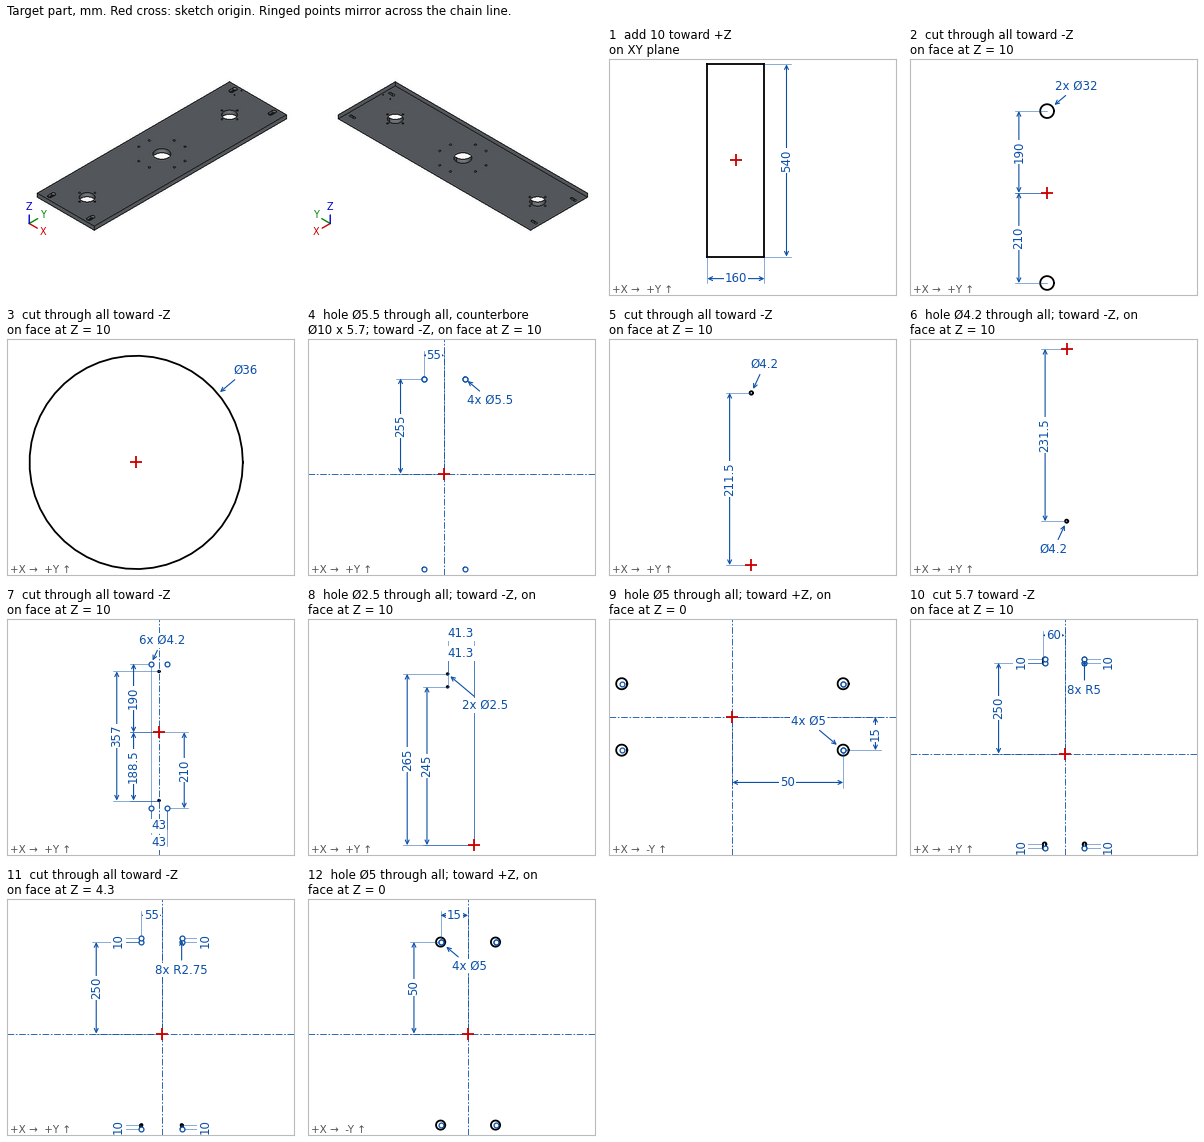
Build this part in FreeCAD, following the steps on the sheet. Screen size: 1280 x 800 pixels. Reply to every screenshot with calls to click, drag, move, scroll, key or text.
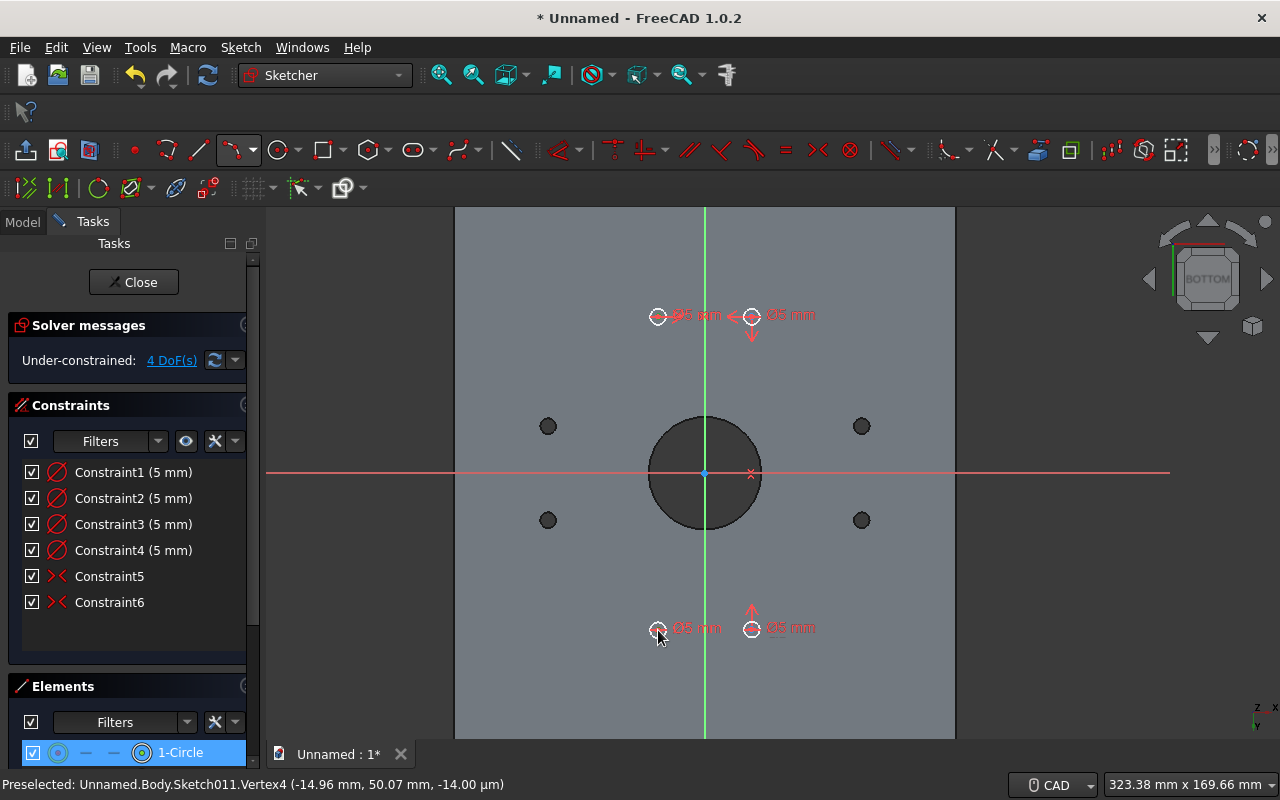
click(353, 473)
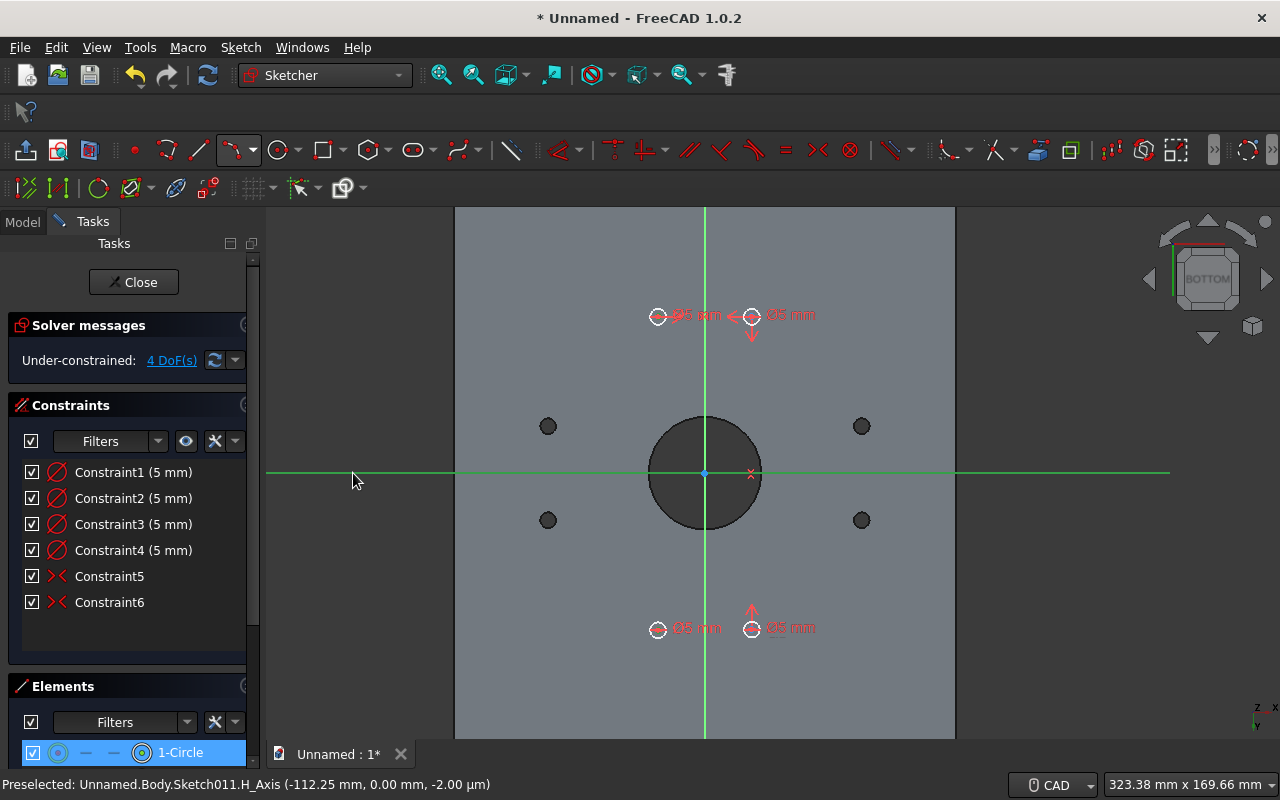
key(s)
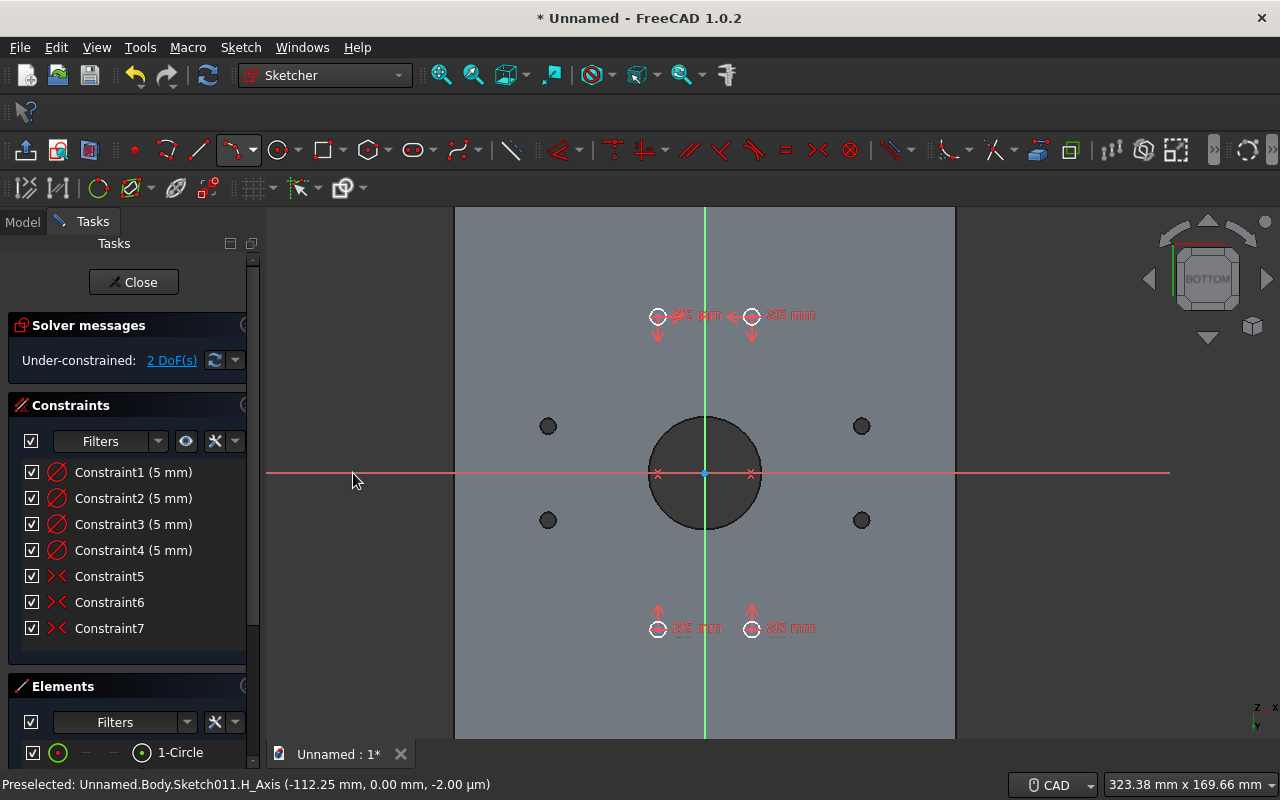
click(558, 150)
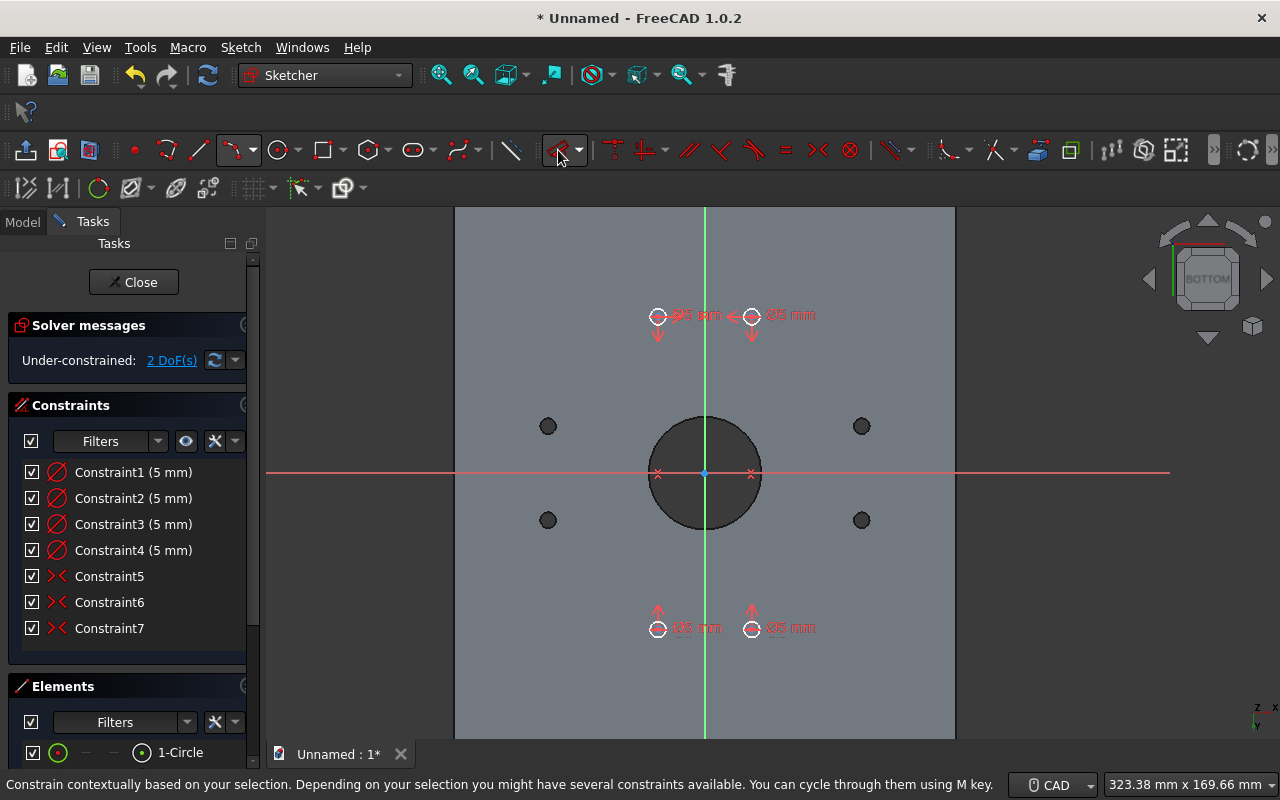
click(658, 317)
click(682, 283)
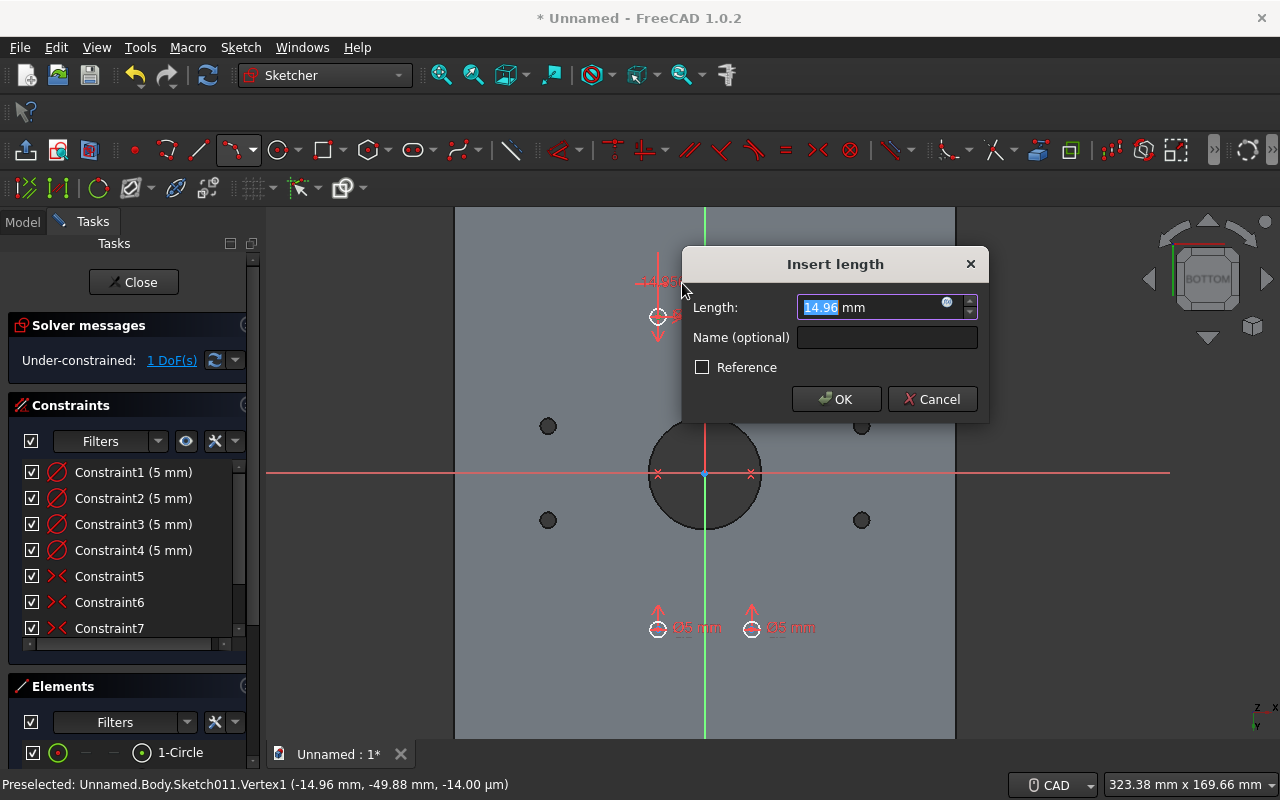
text(15)
key(Return)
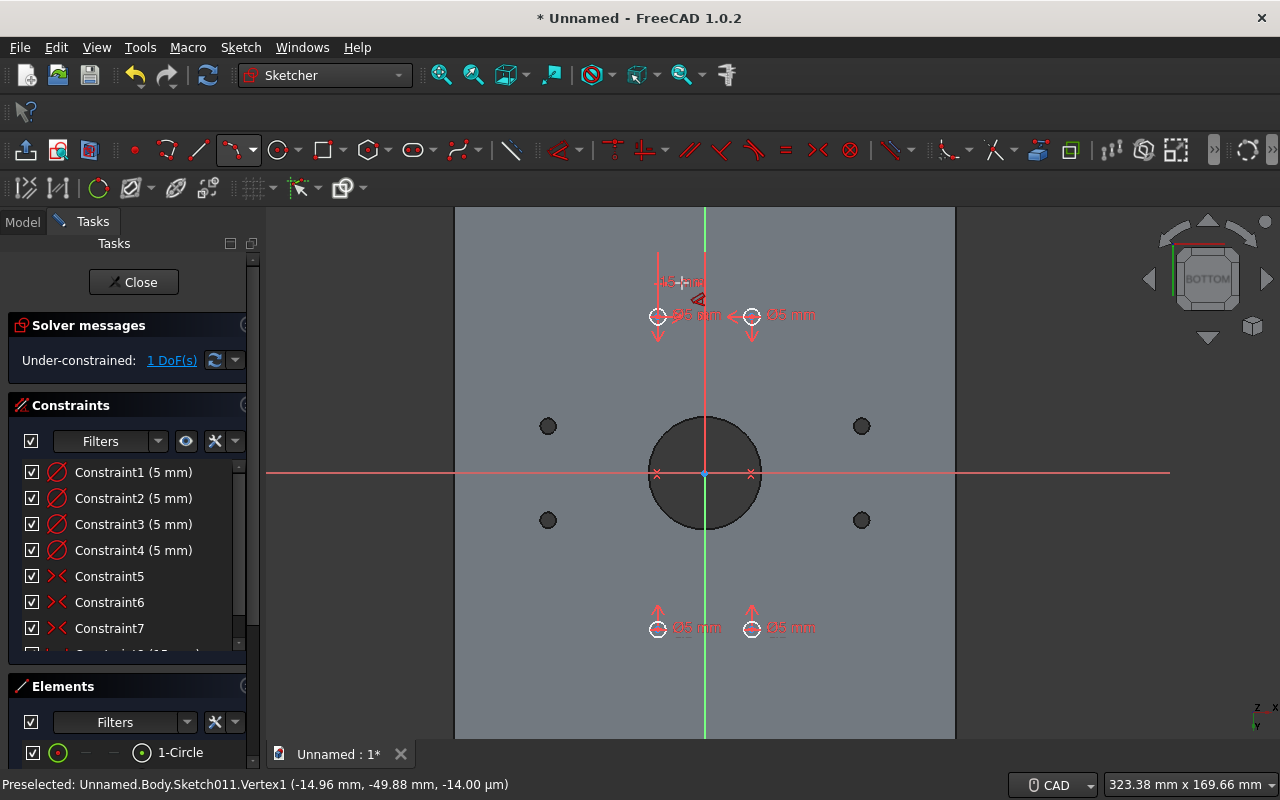
click(658, 317)
click(624, 395)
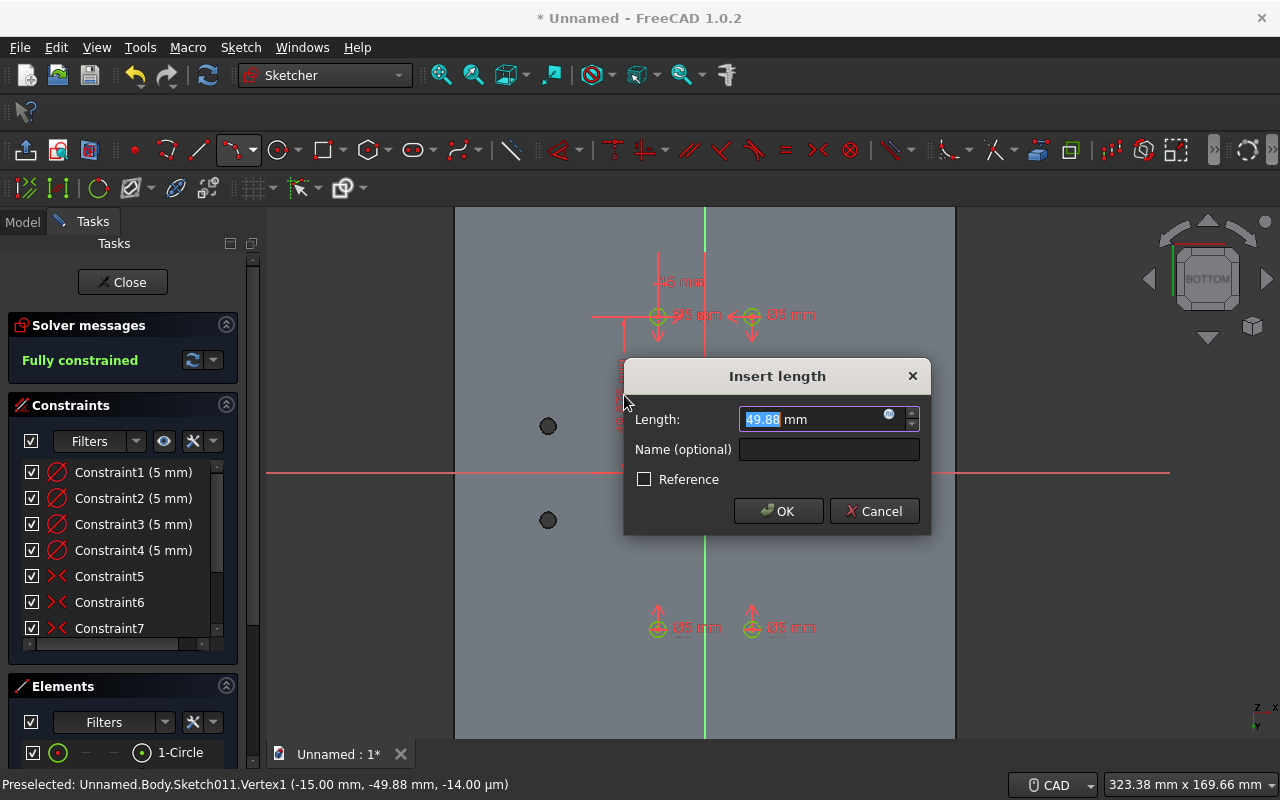
text(50)
key(Return)
key(Escape)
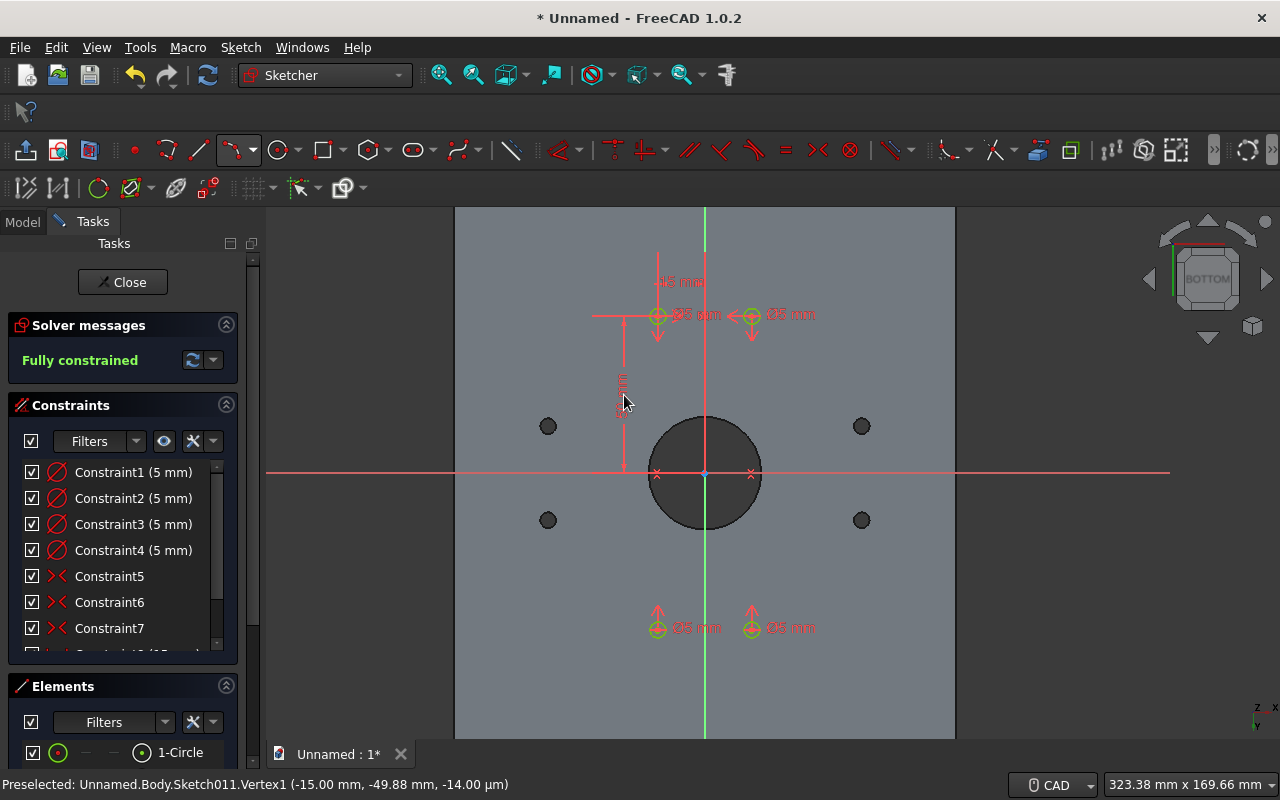
click(123, 282)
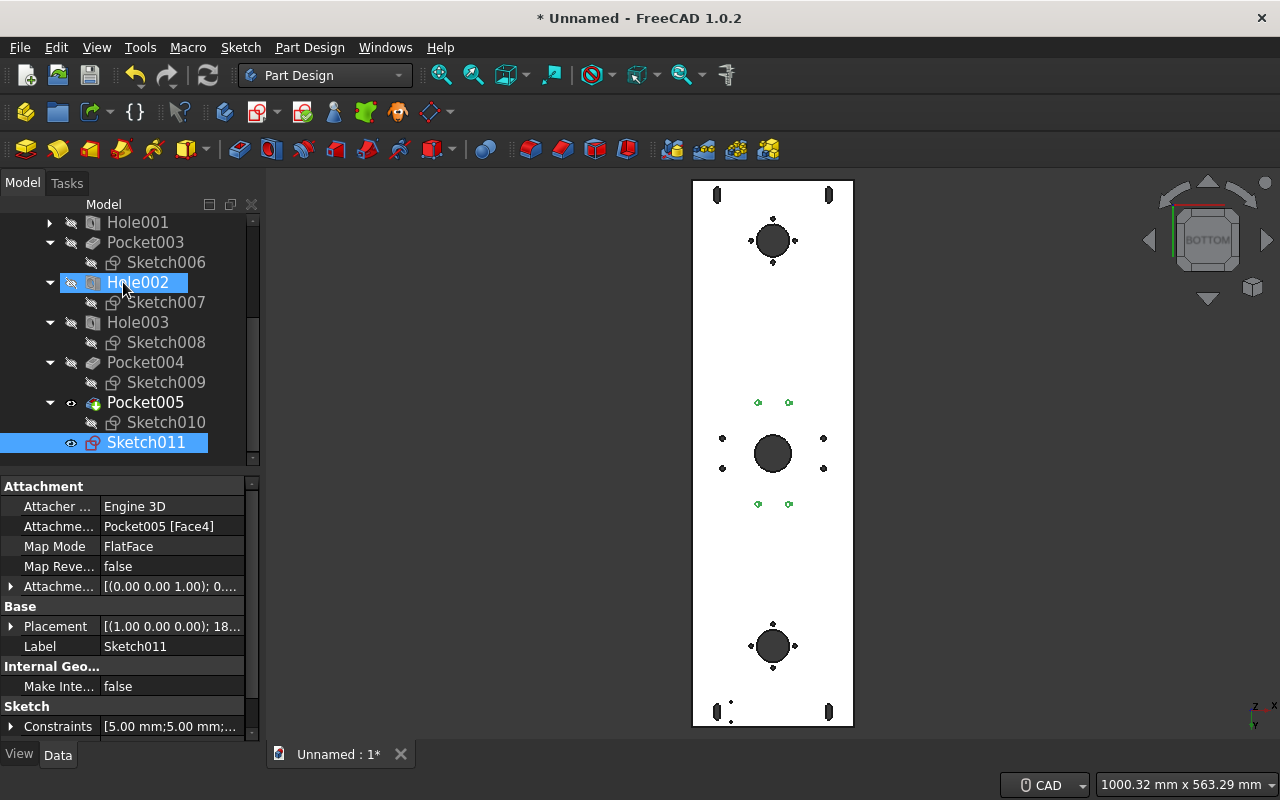
click(272, 150)